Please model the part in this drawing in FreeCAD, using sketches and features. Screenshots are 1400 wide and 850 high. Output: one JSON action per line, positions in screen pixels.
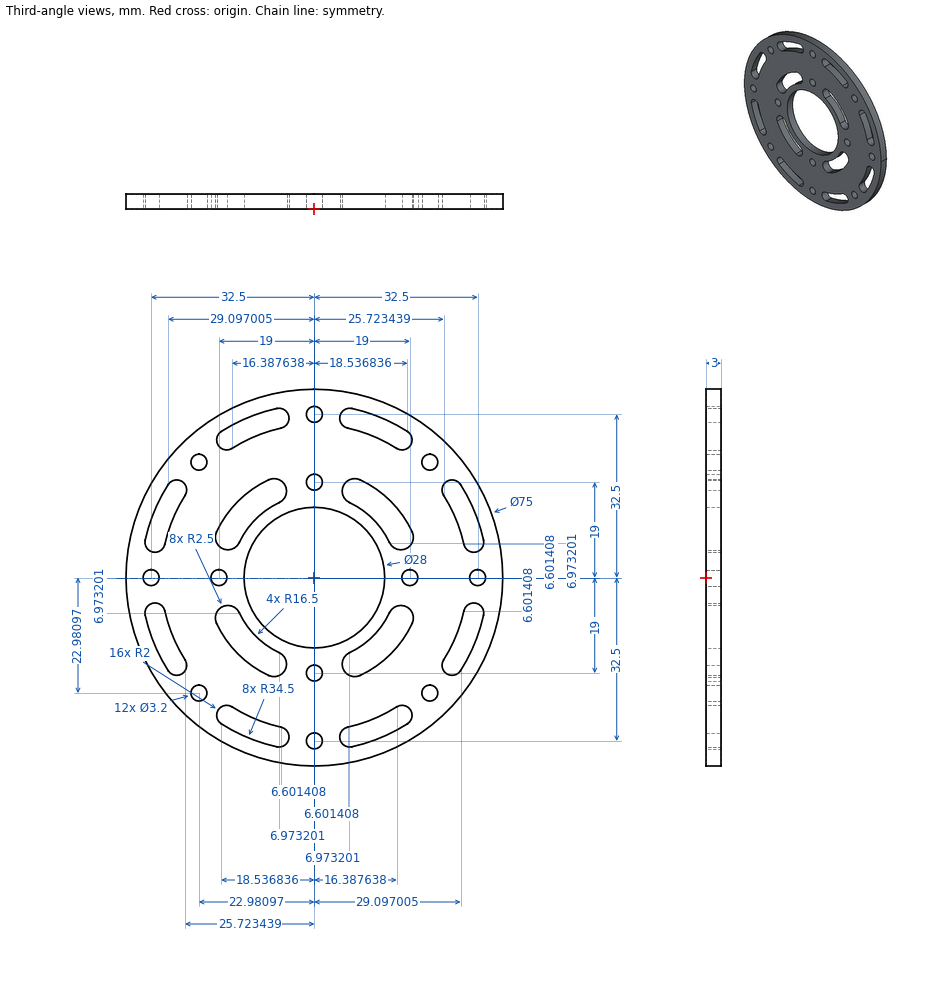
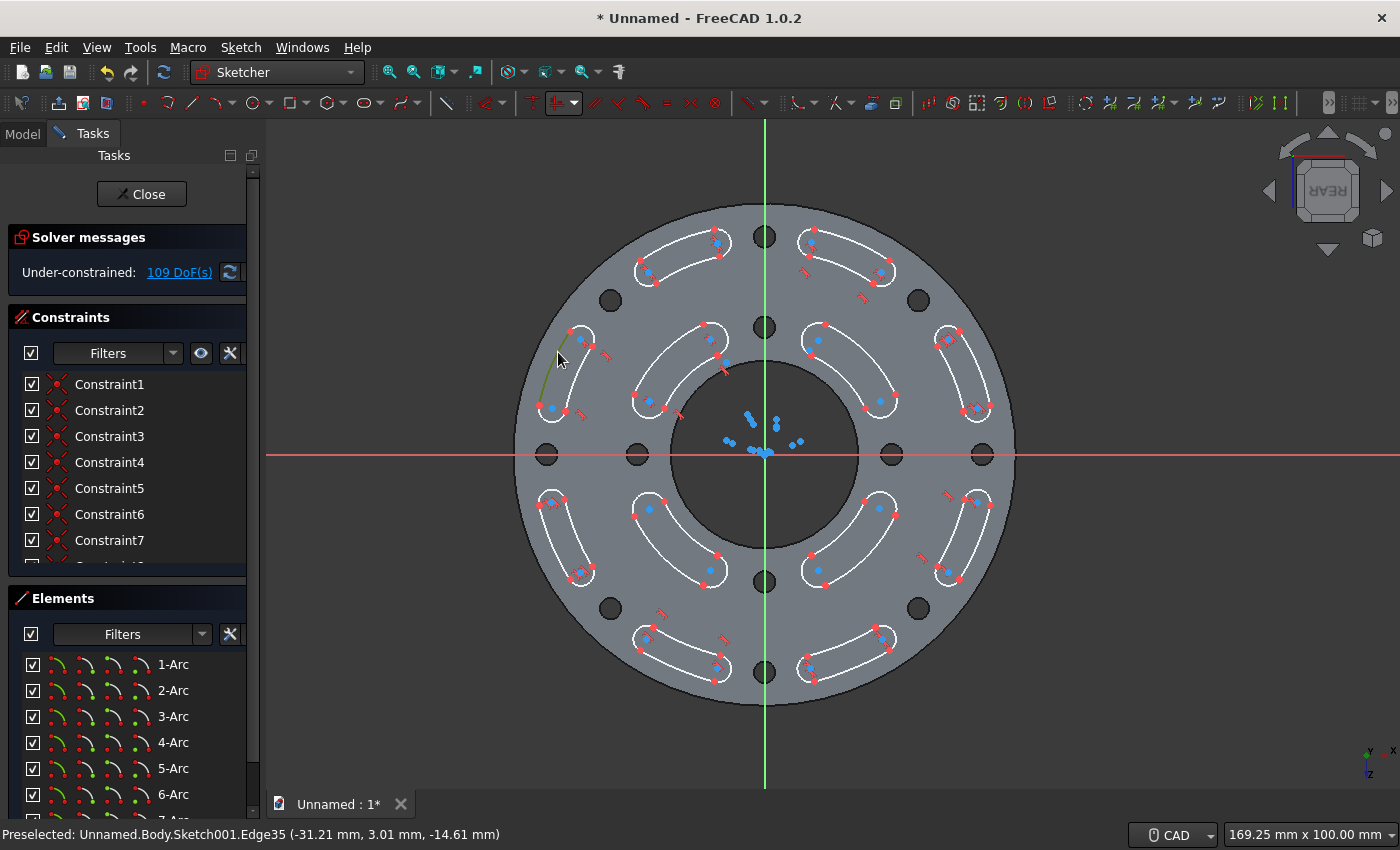
{"action": "left_click", "coordinate": [542, 418]}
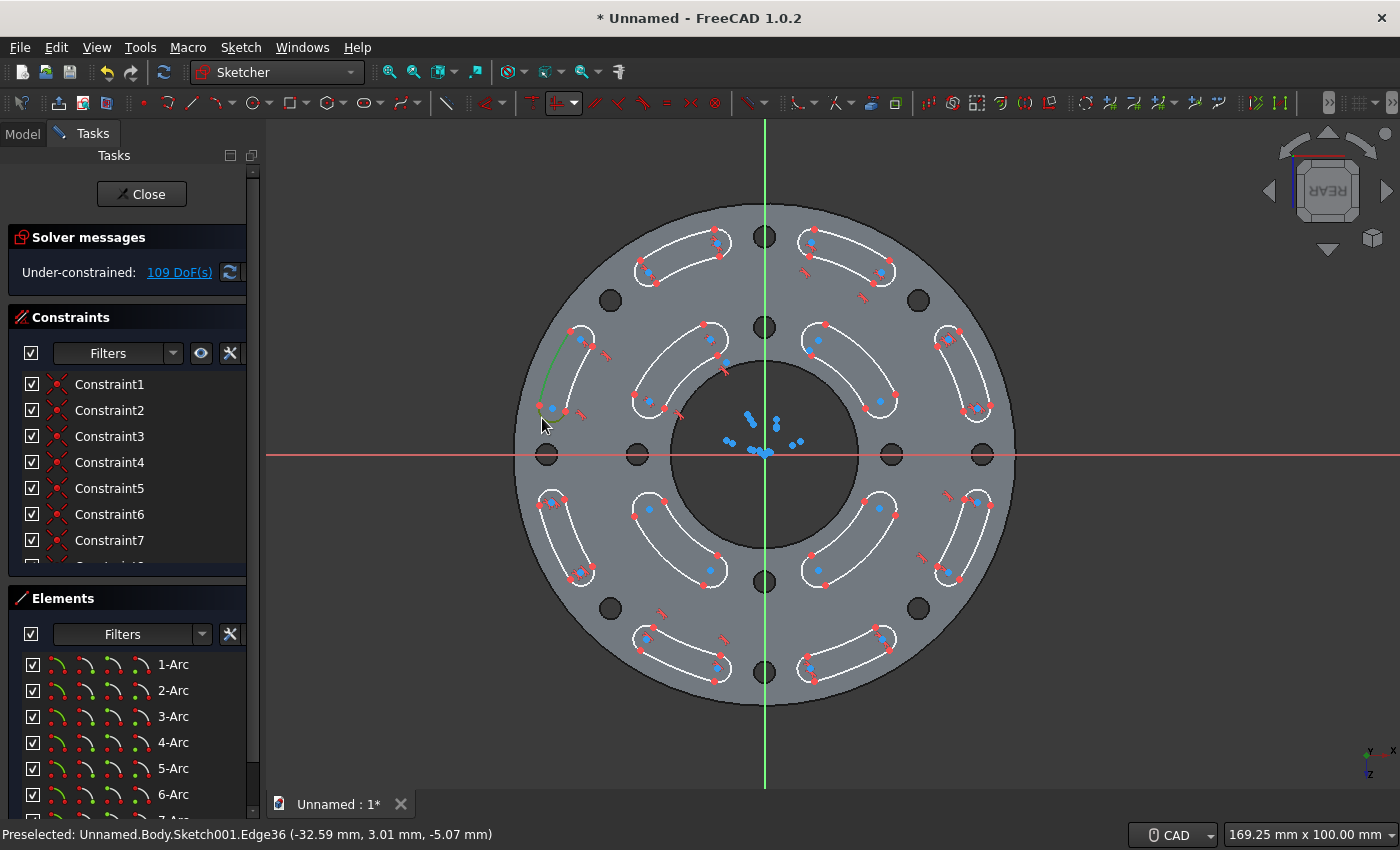
{"action": "left_click", "coordinate": [644, 104]}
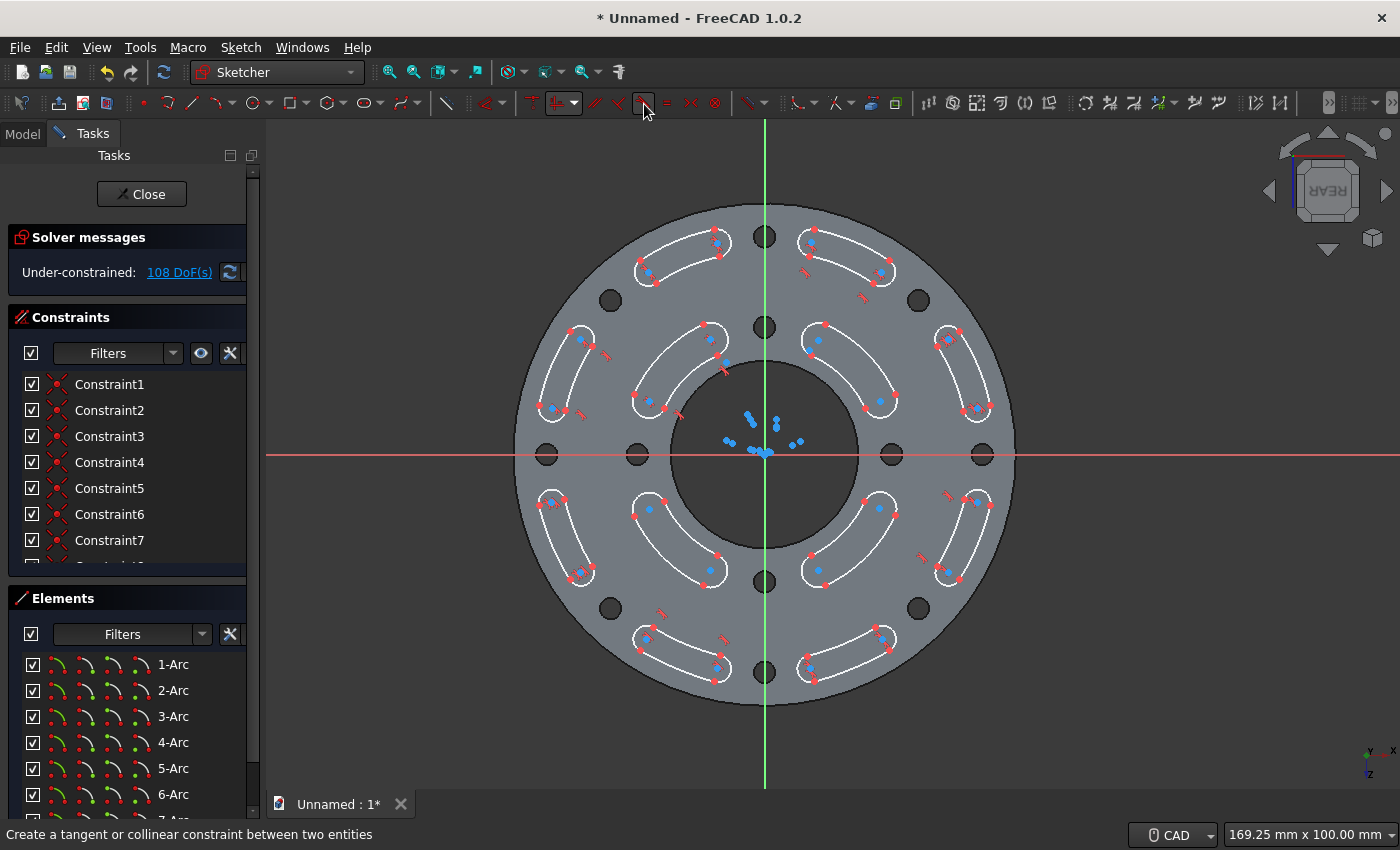
{"action": "left_click", "coordinate": [853, 389]}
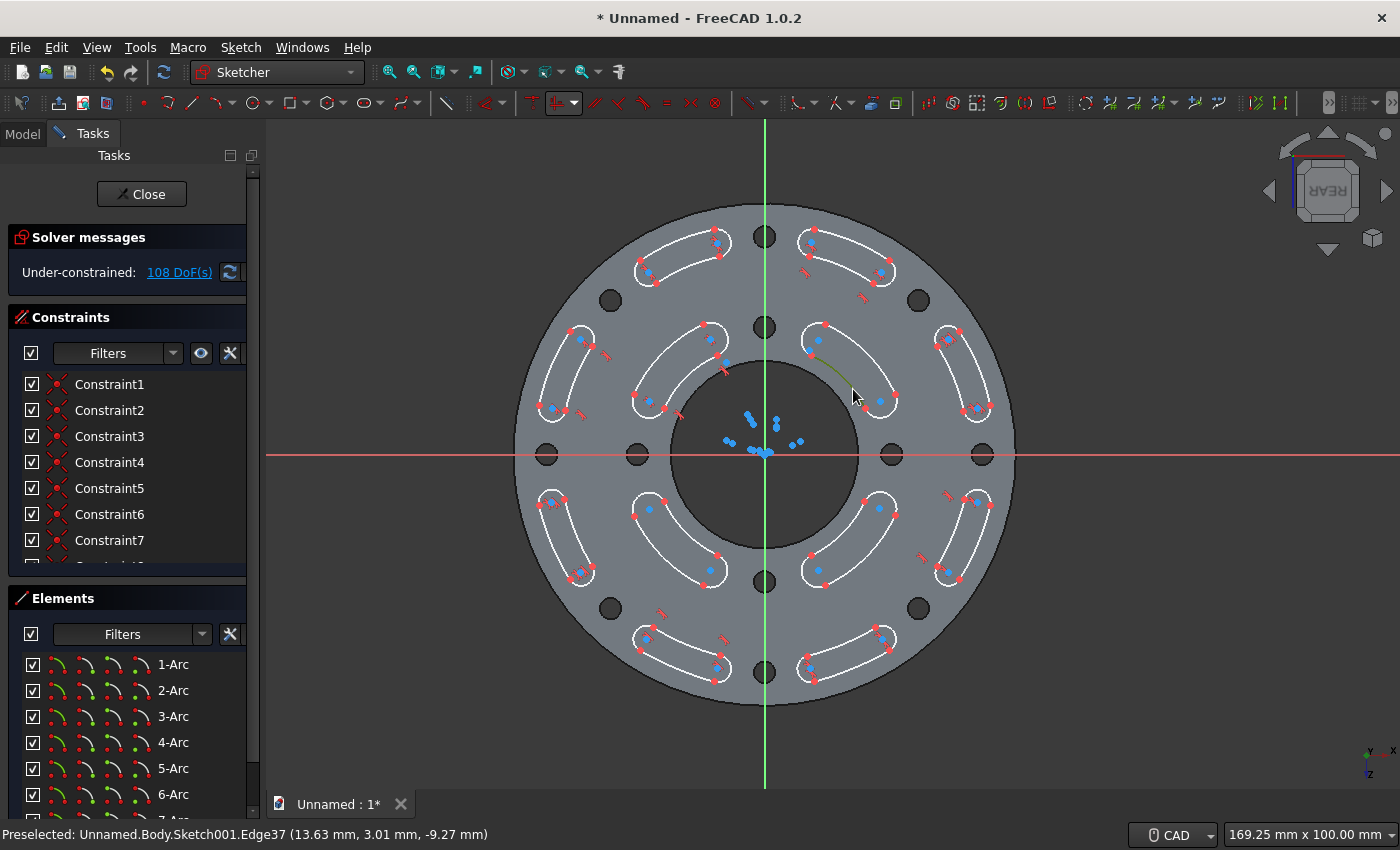
{"action": "left_click", "coordinate": [877, 418]}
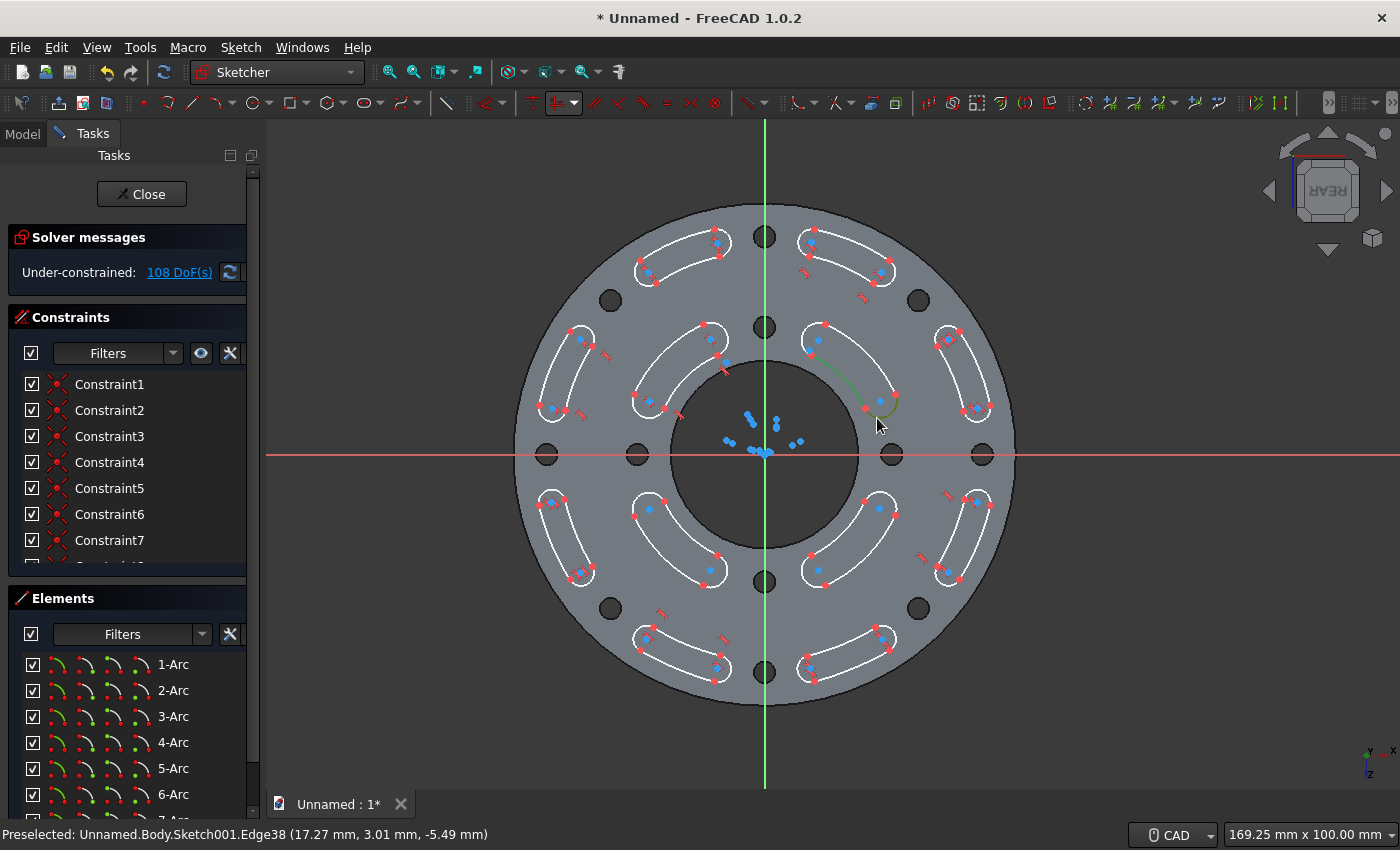
{"action": "left_click", "coordinate": [644, 104]}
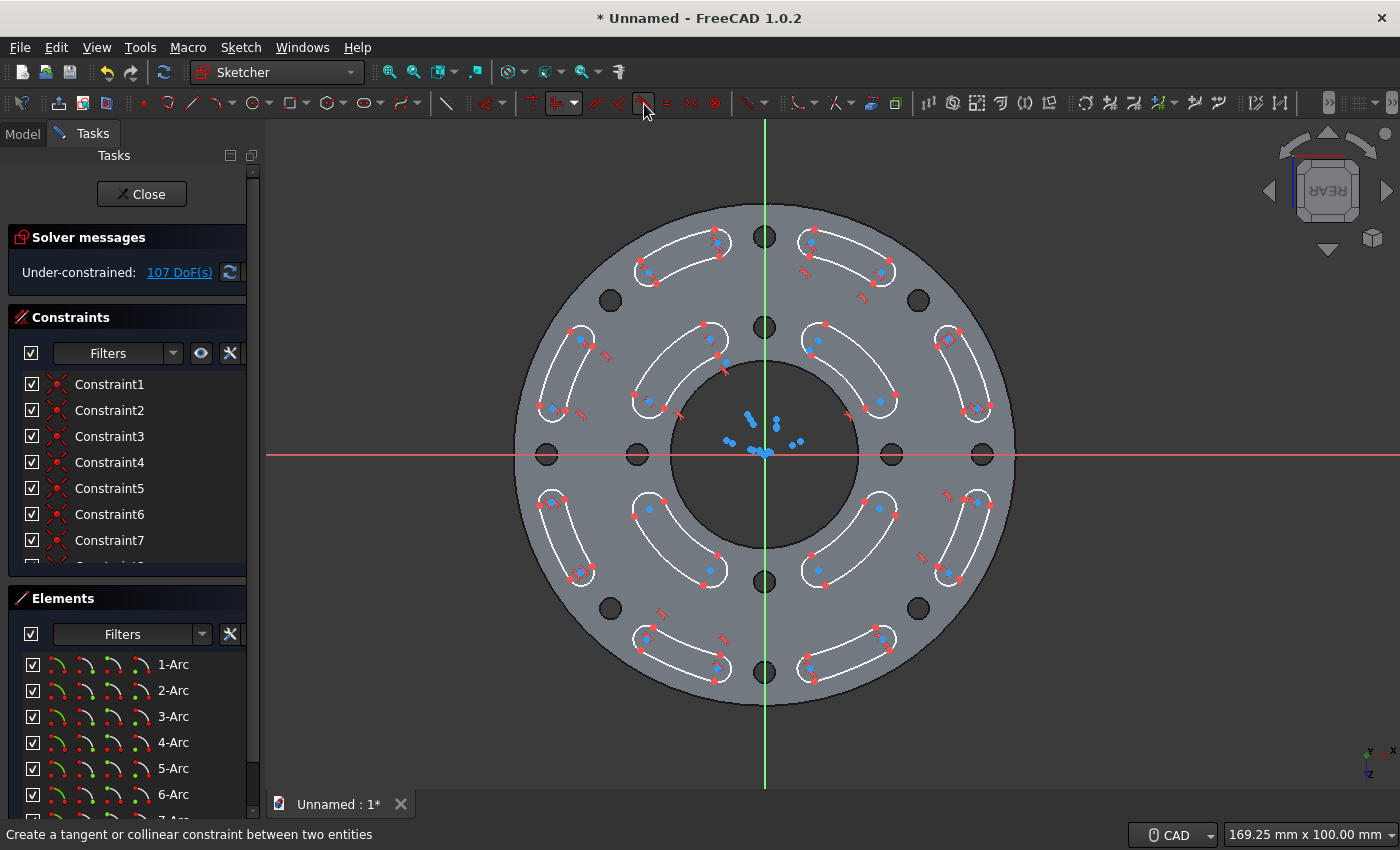
{"action": "left_click", "coordinate": [853, 388]}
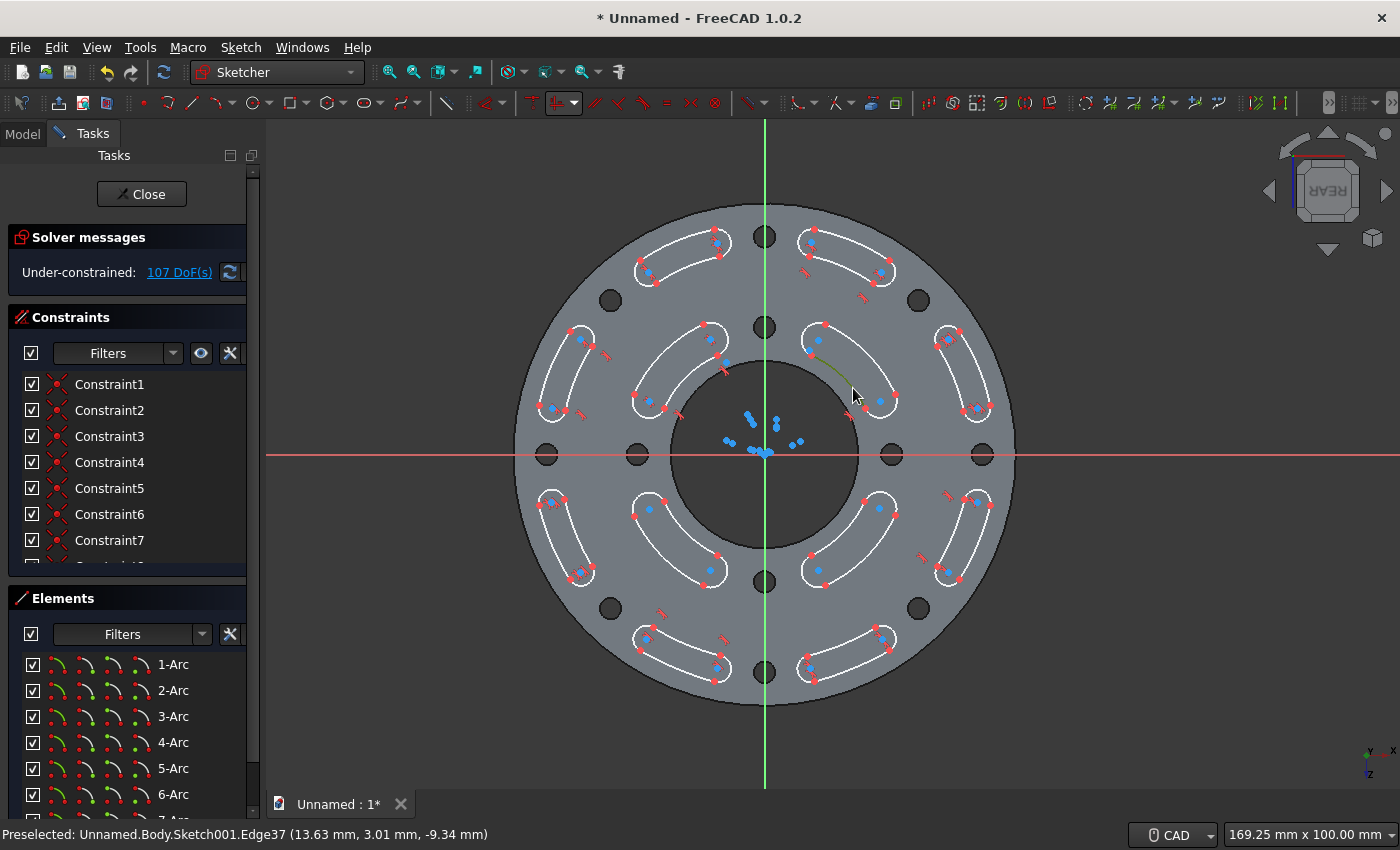
{"action": "left_click", "coordinate": [810, 325]}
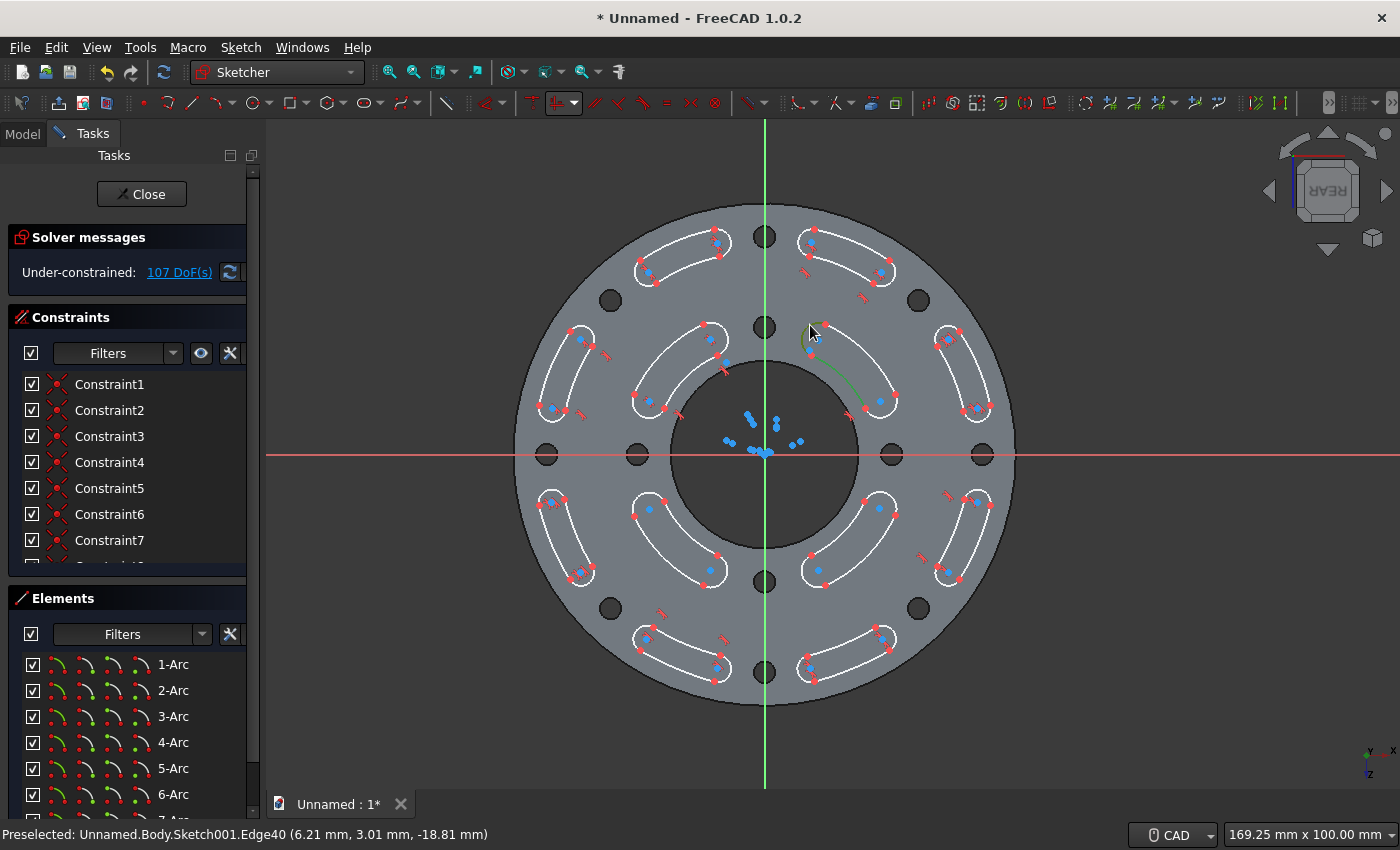
{"action": "left_click", "coordinate": [644, 104]}